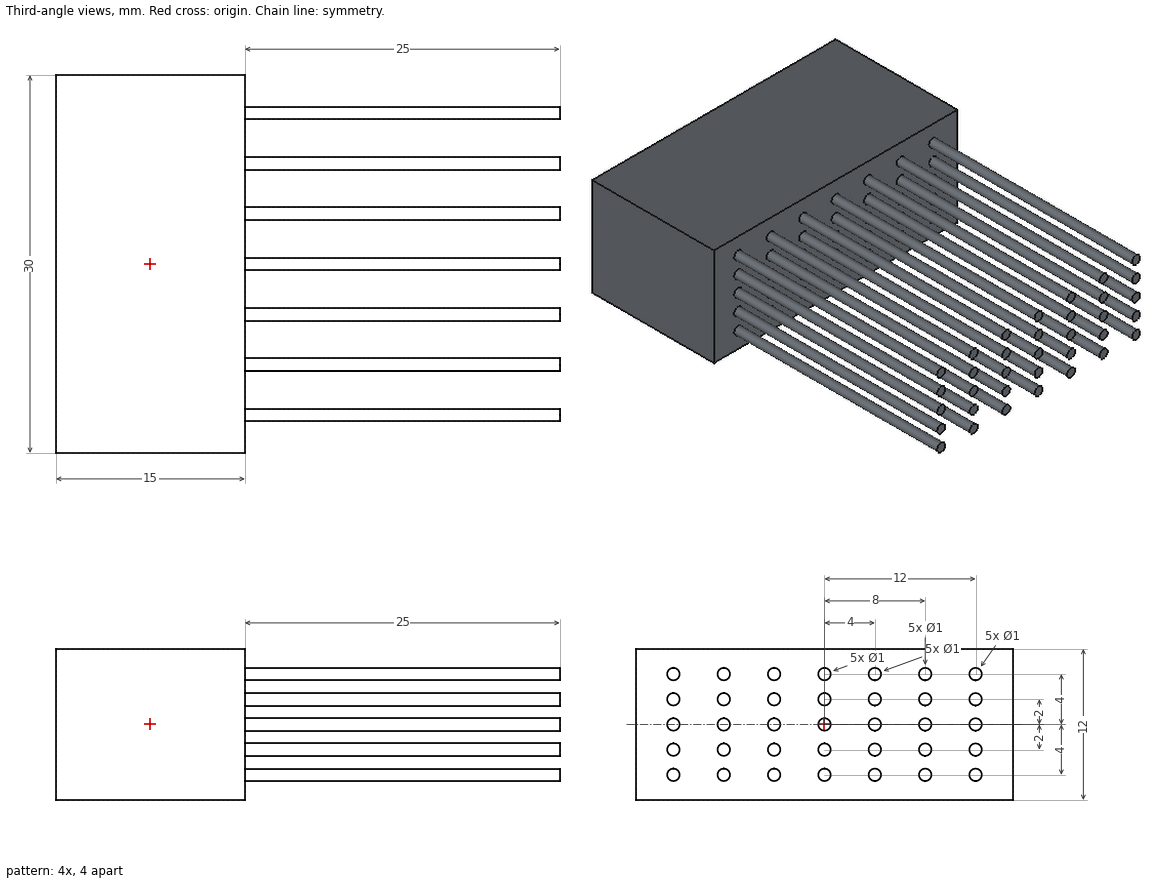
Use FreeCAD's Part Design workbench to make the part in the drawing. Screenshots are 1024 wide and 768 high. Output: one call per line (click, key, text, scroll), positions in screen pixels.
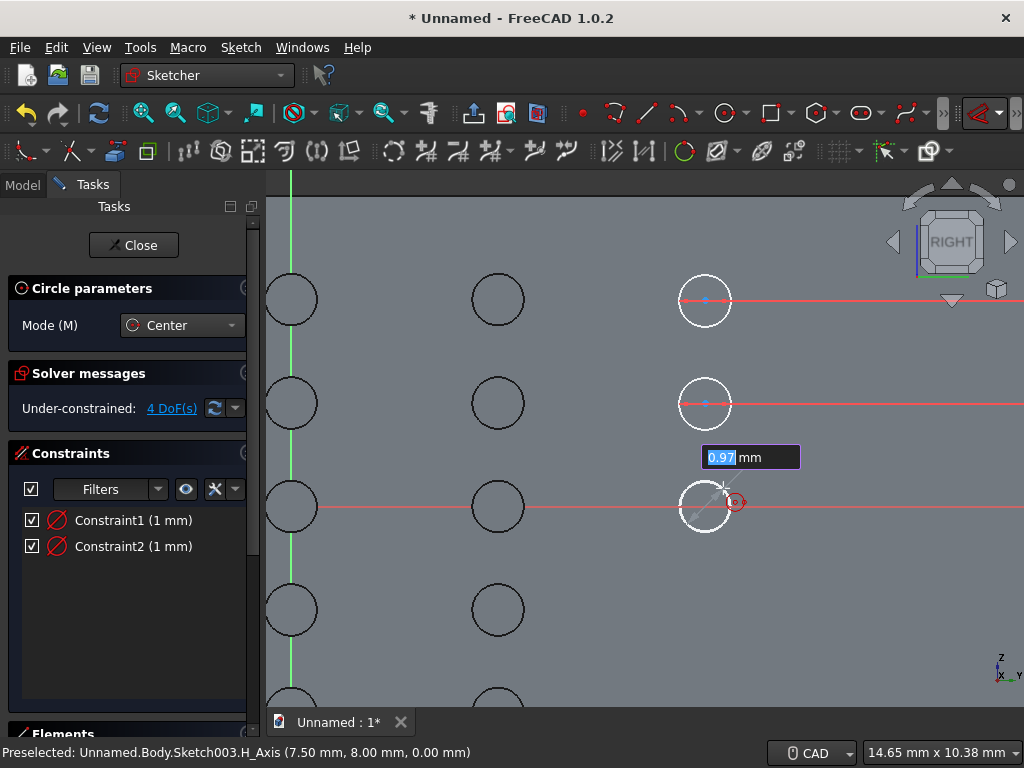
text(1)
key(Return)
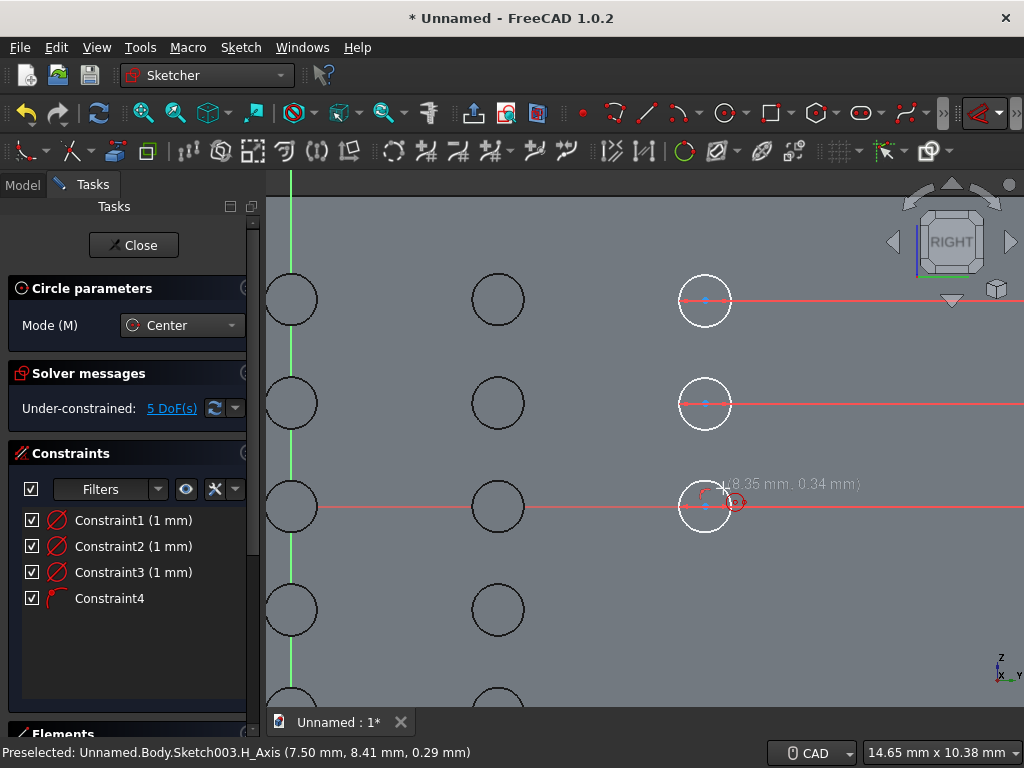
click(705, 610)
move(723, 592)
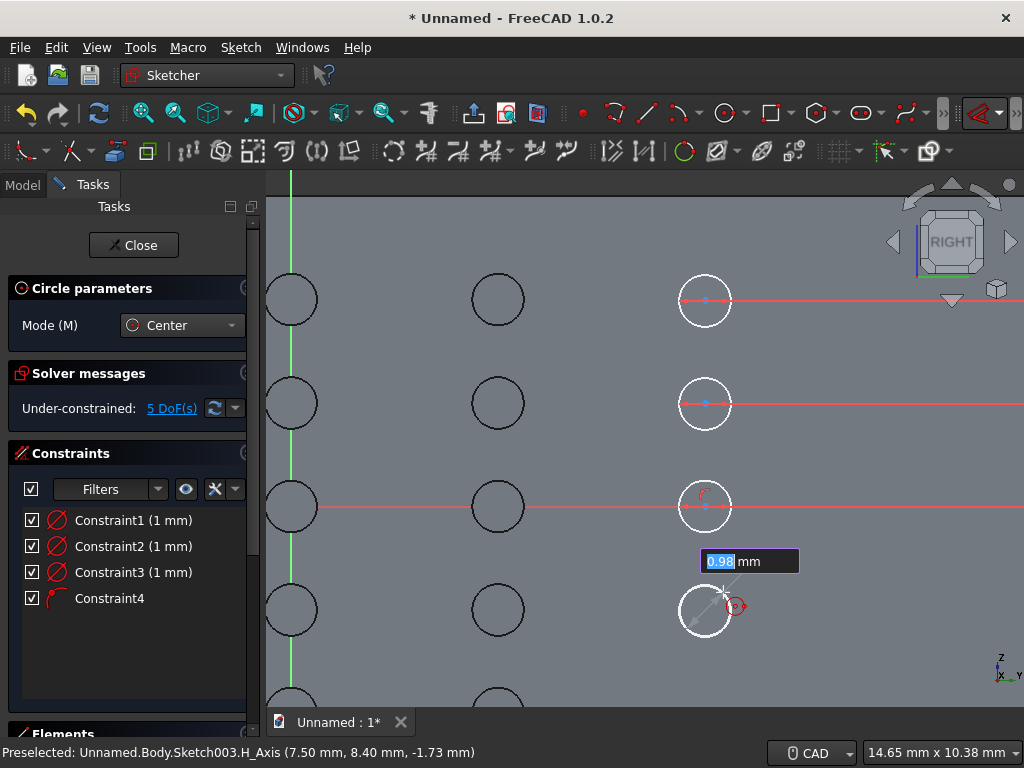
text(1)
key(Return)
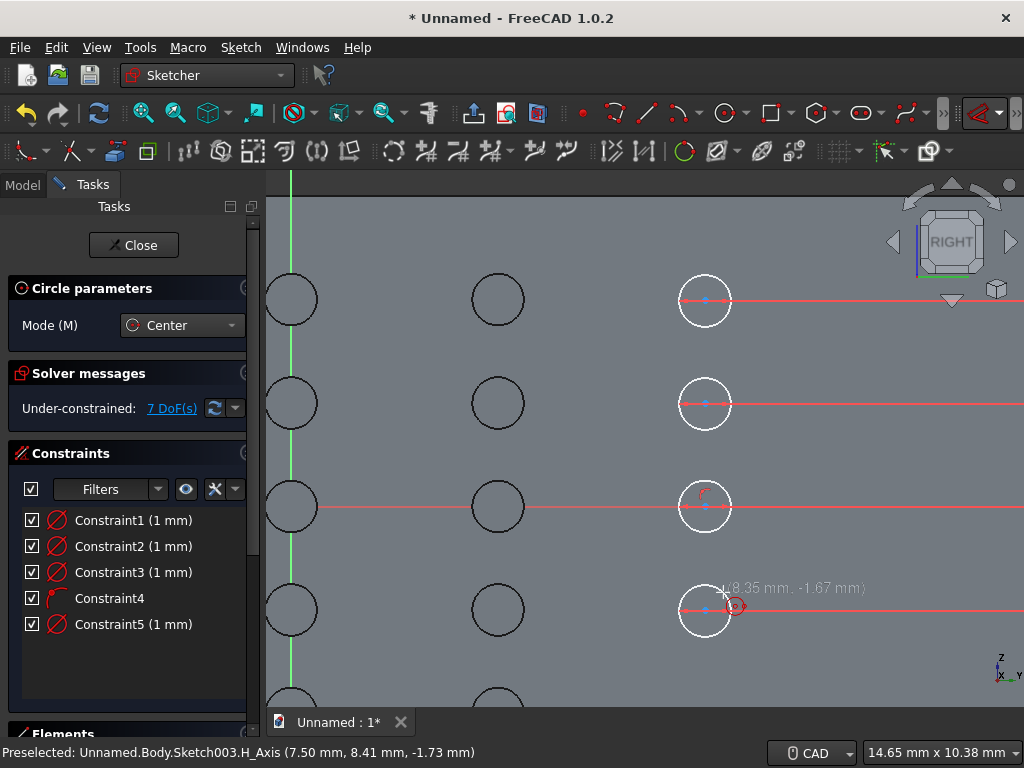
scroll(710, 300, down, 2)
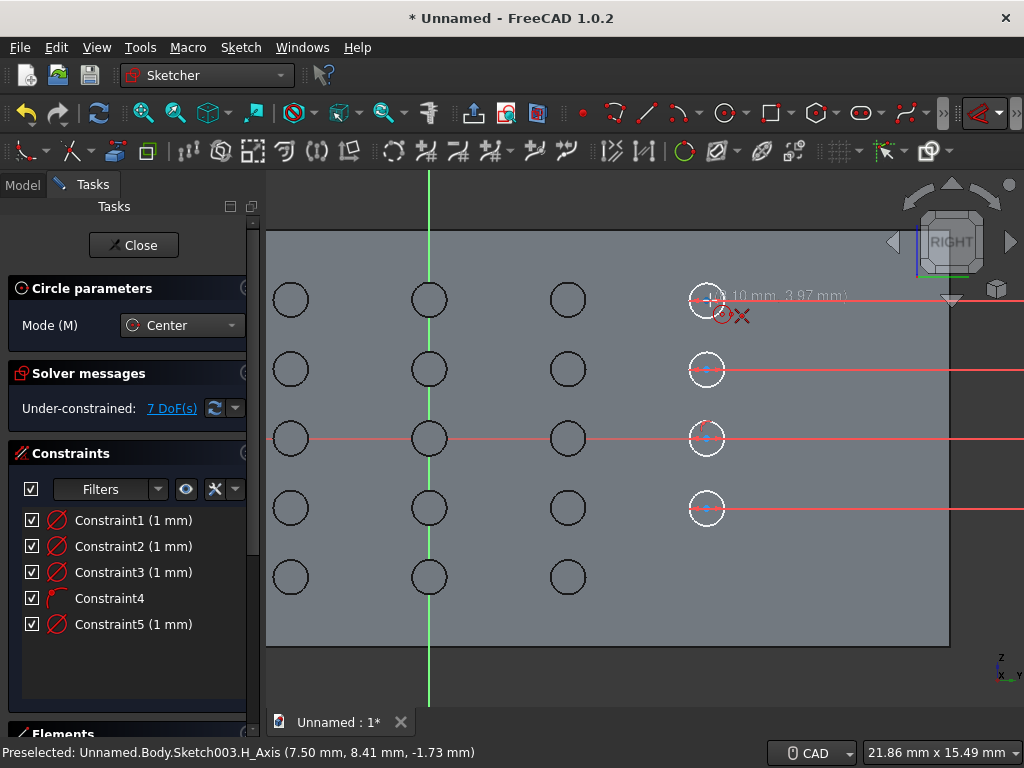
scroll(707, 577, up, 2)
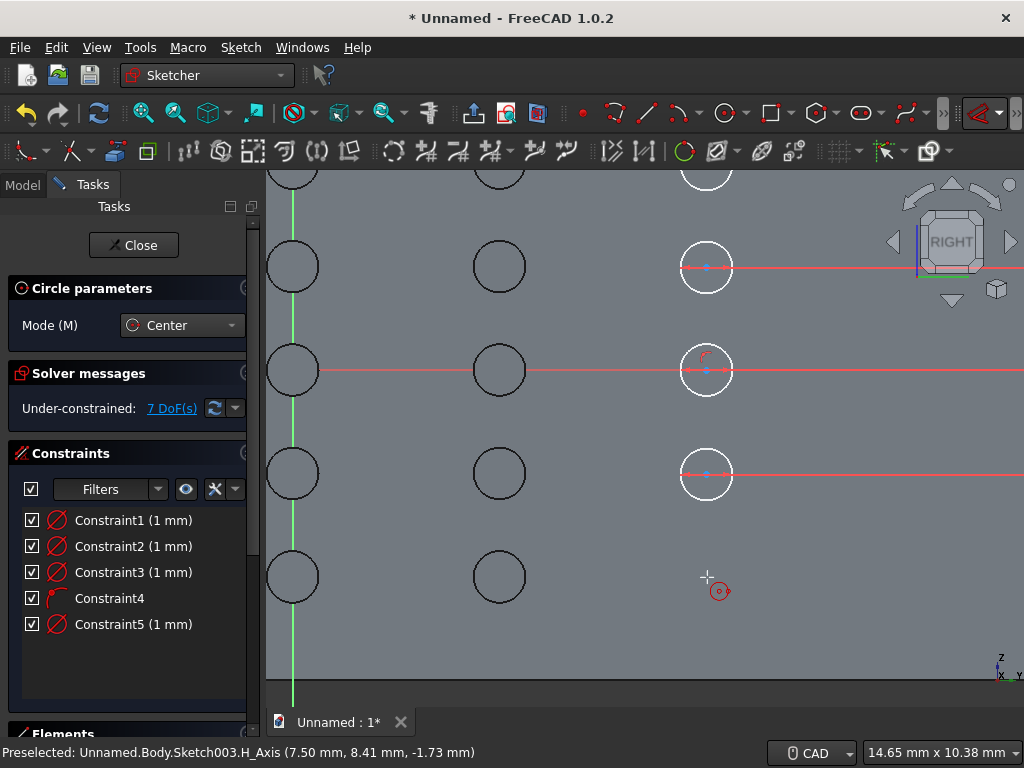
click(706, 577)
move(725, 559)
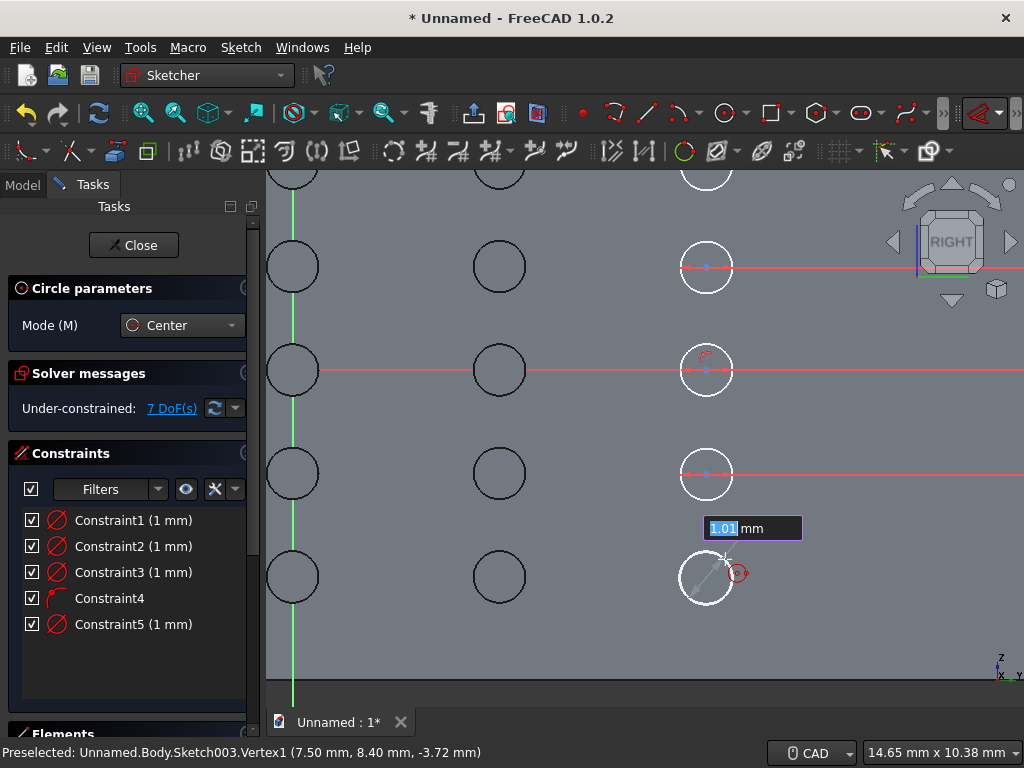
text(1)
key(Return)
key(Escape)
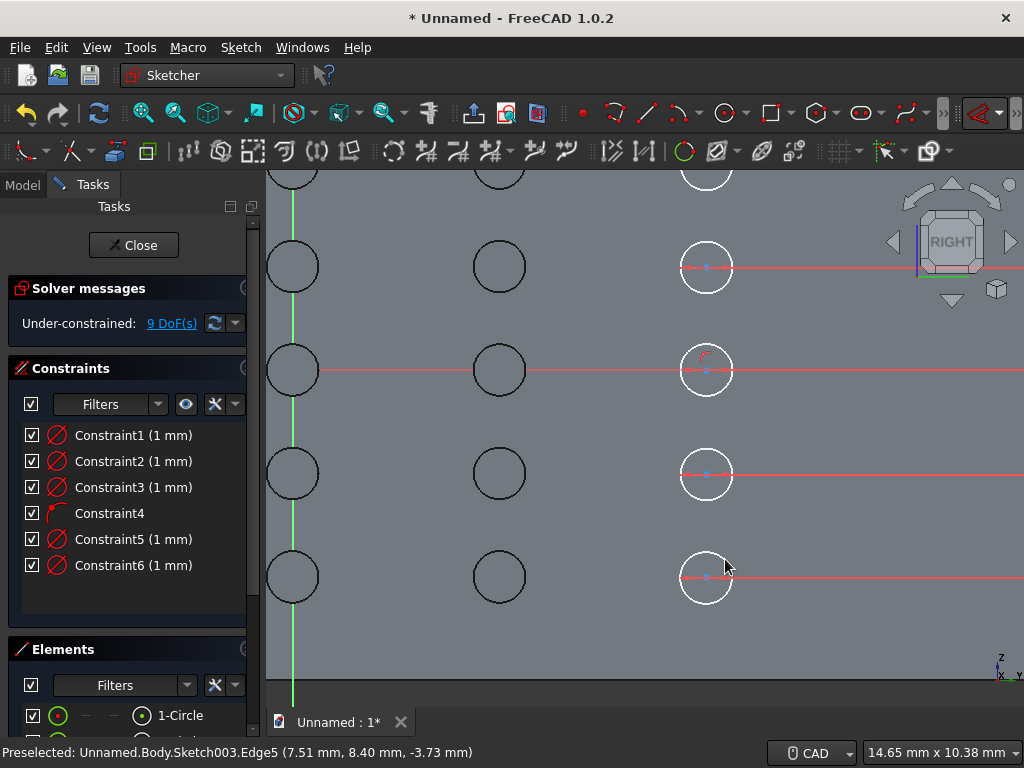
click(706, 268)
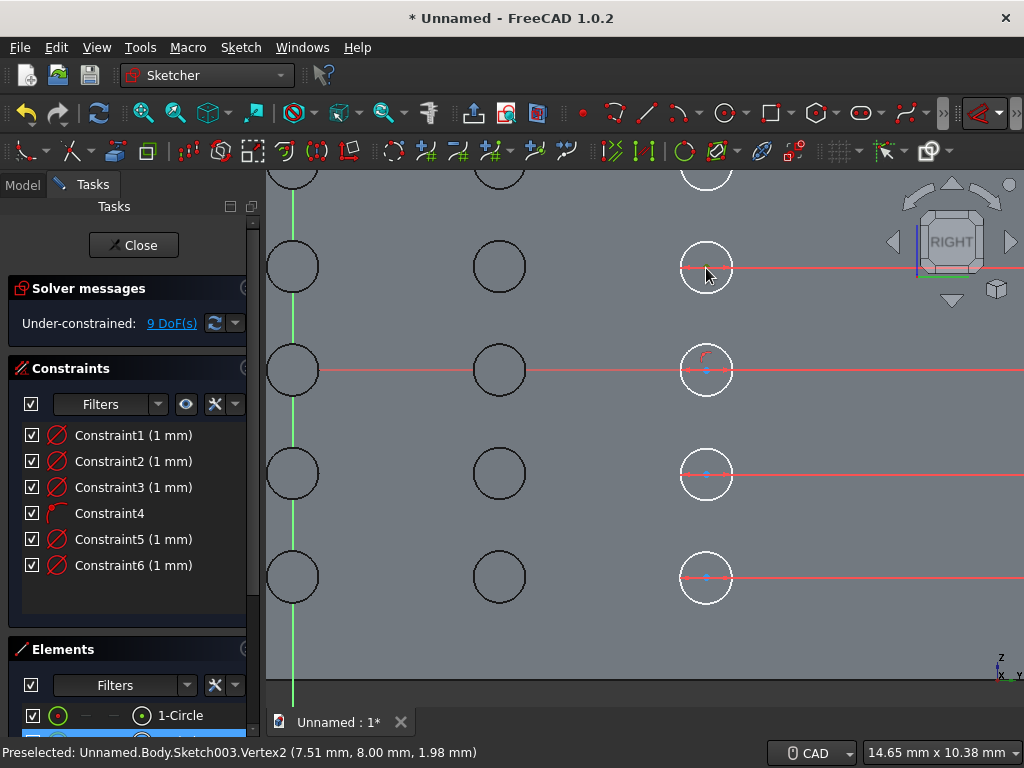
click(706, 475)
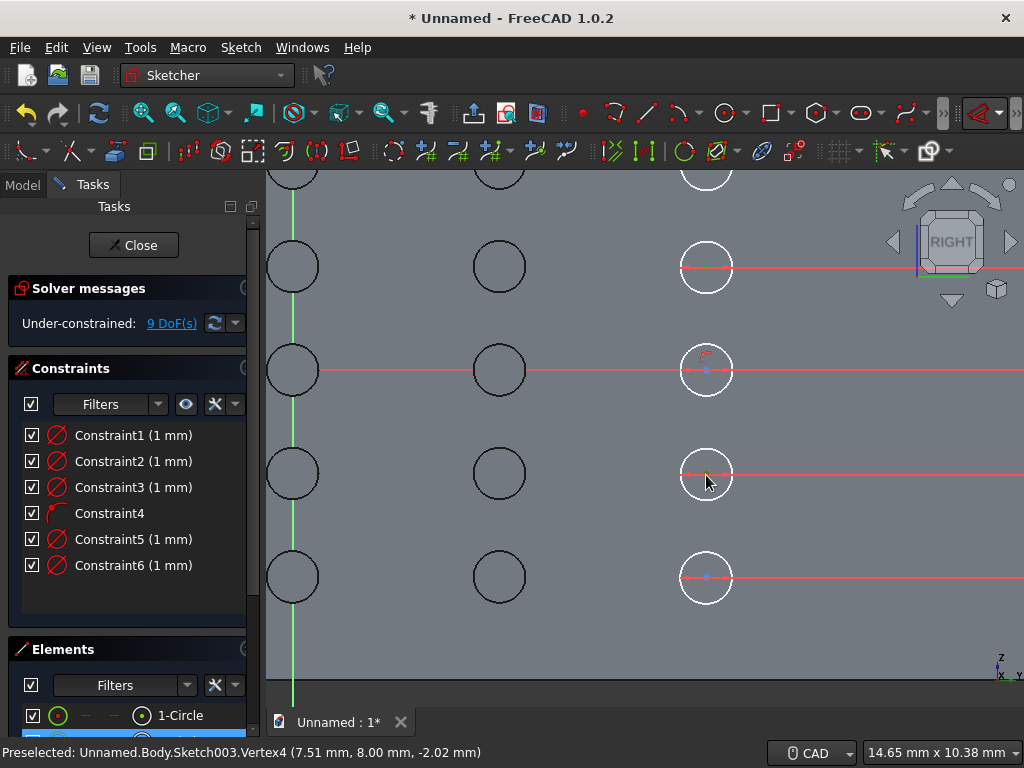
click(334, 370)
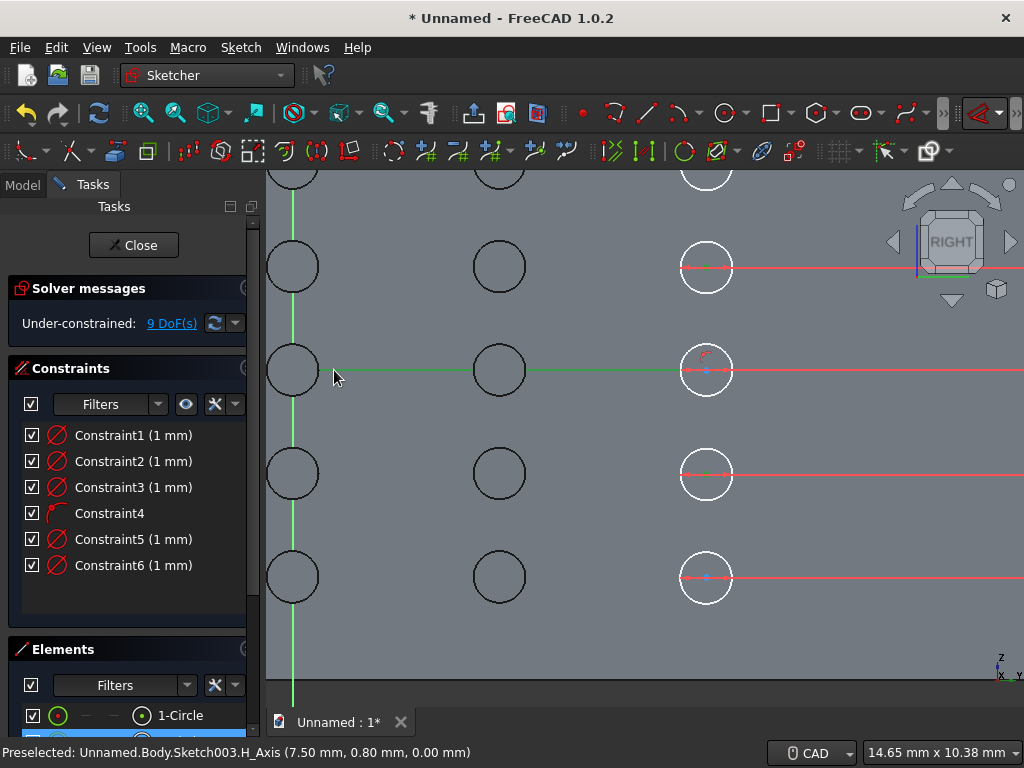
key(s)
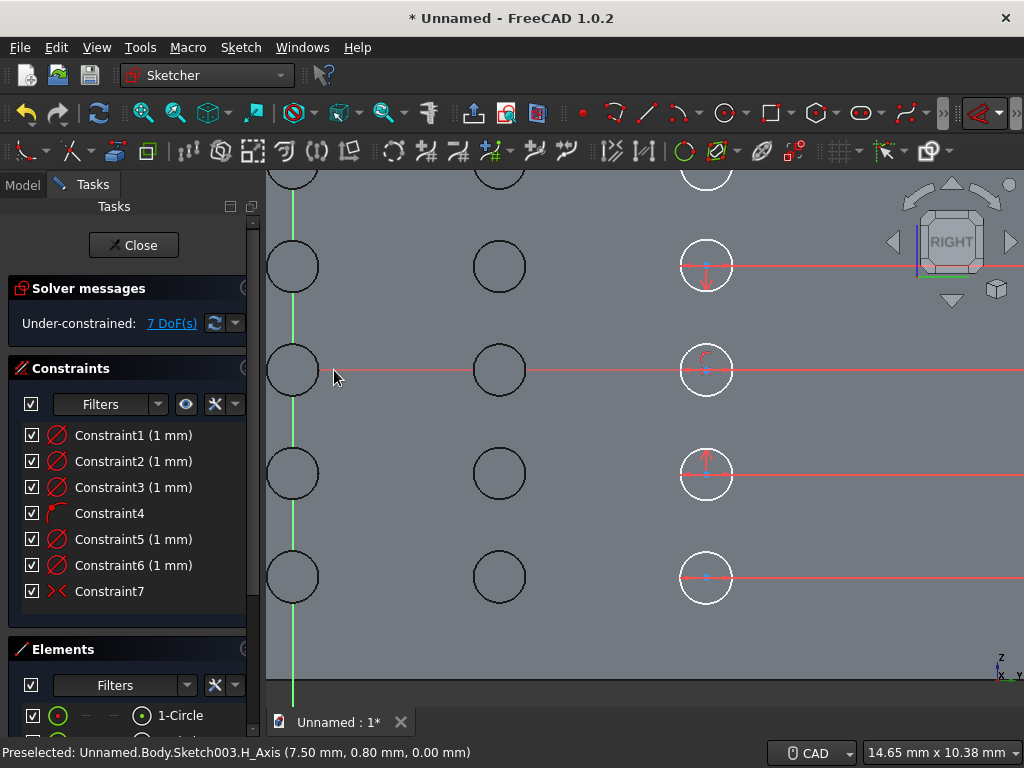
scroll(707, 578, down, 2)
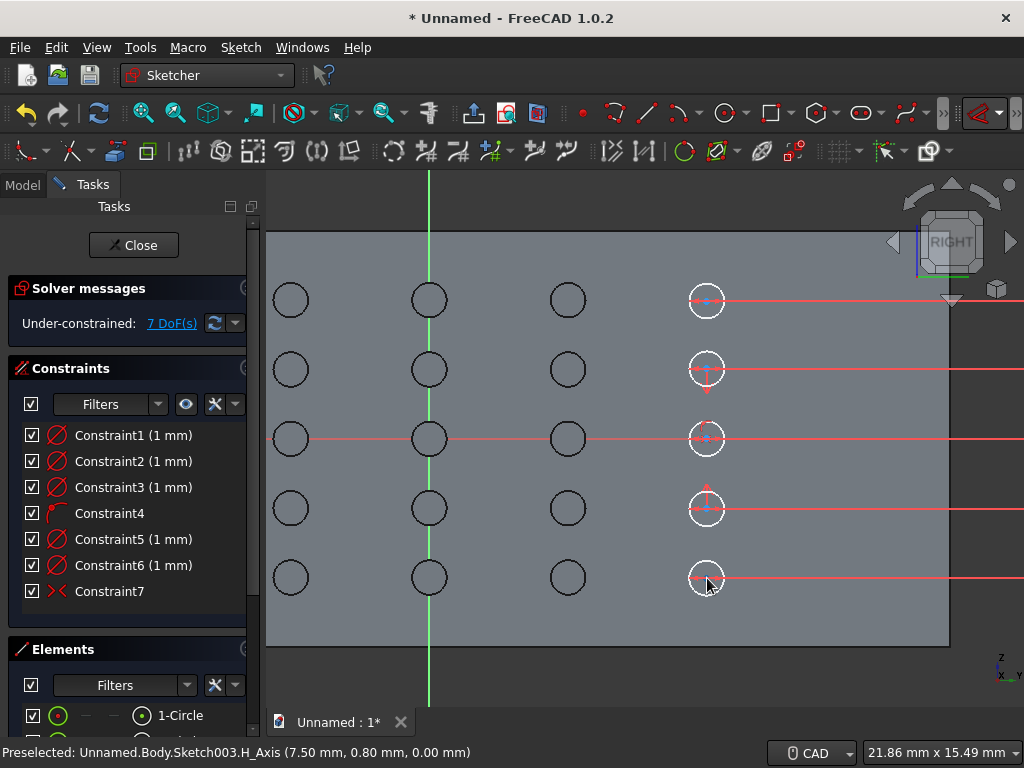
click(707, 301)